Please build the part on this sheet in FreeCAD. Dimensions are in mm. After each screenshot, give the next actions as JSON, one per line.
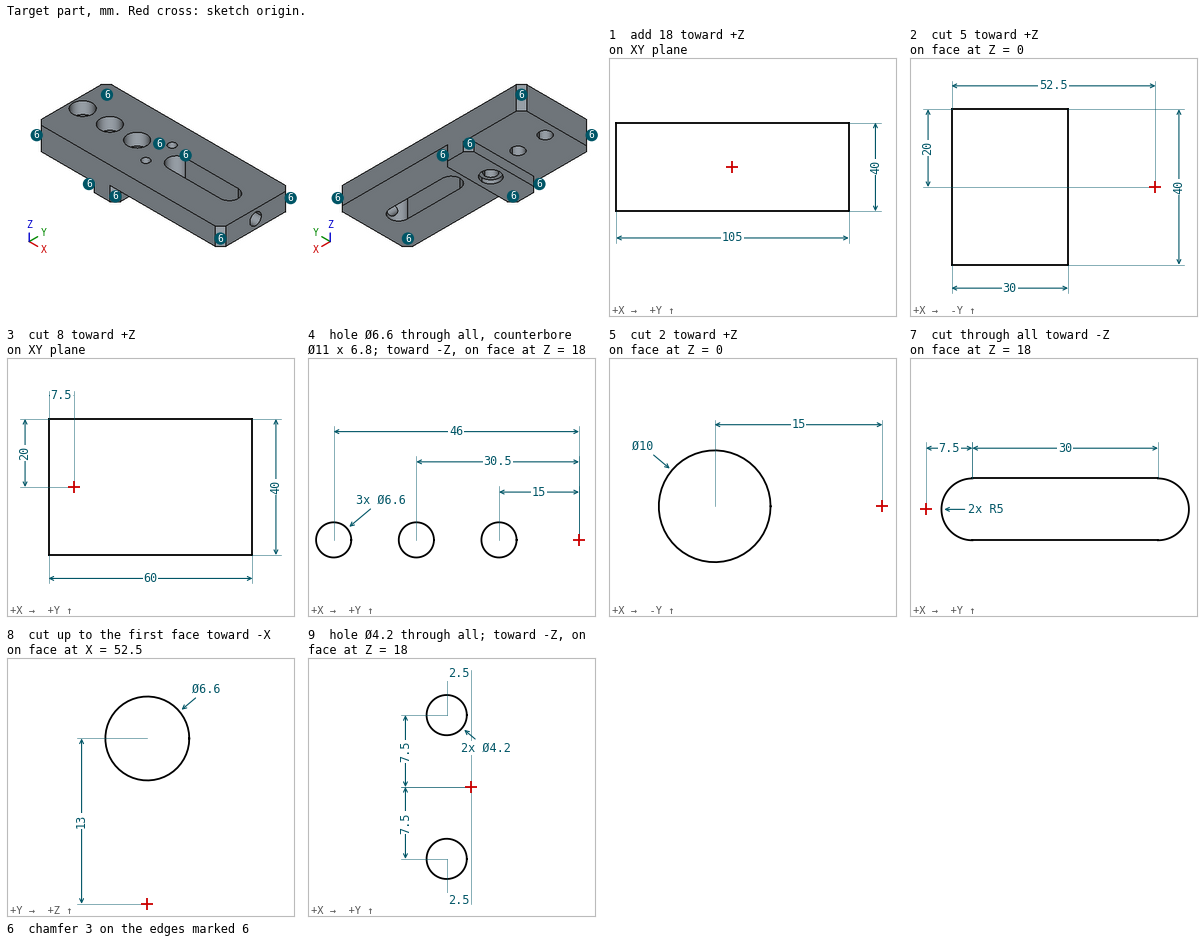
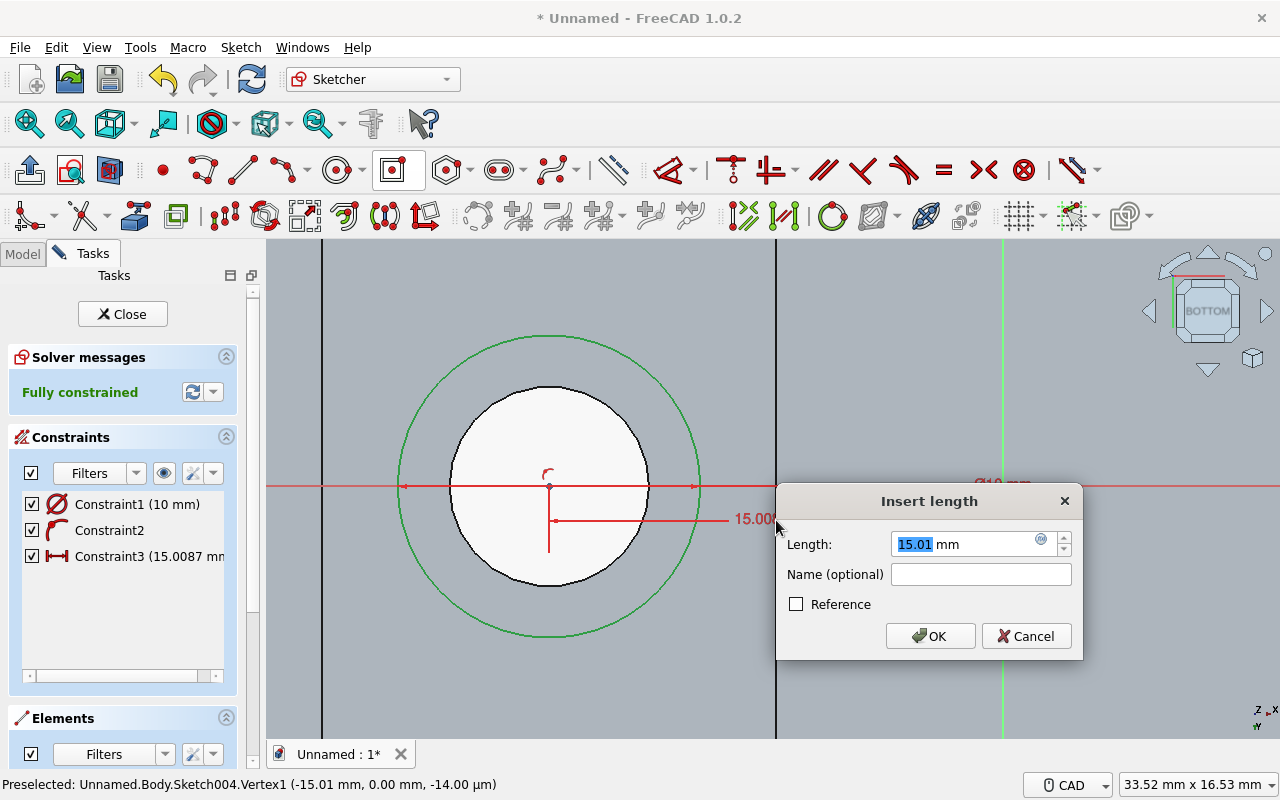
{"action": "type", "text": "15"}
{"action": "key", "text": "Return"}
{"action": "key", "text": "Escape"}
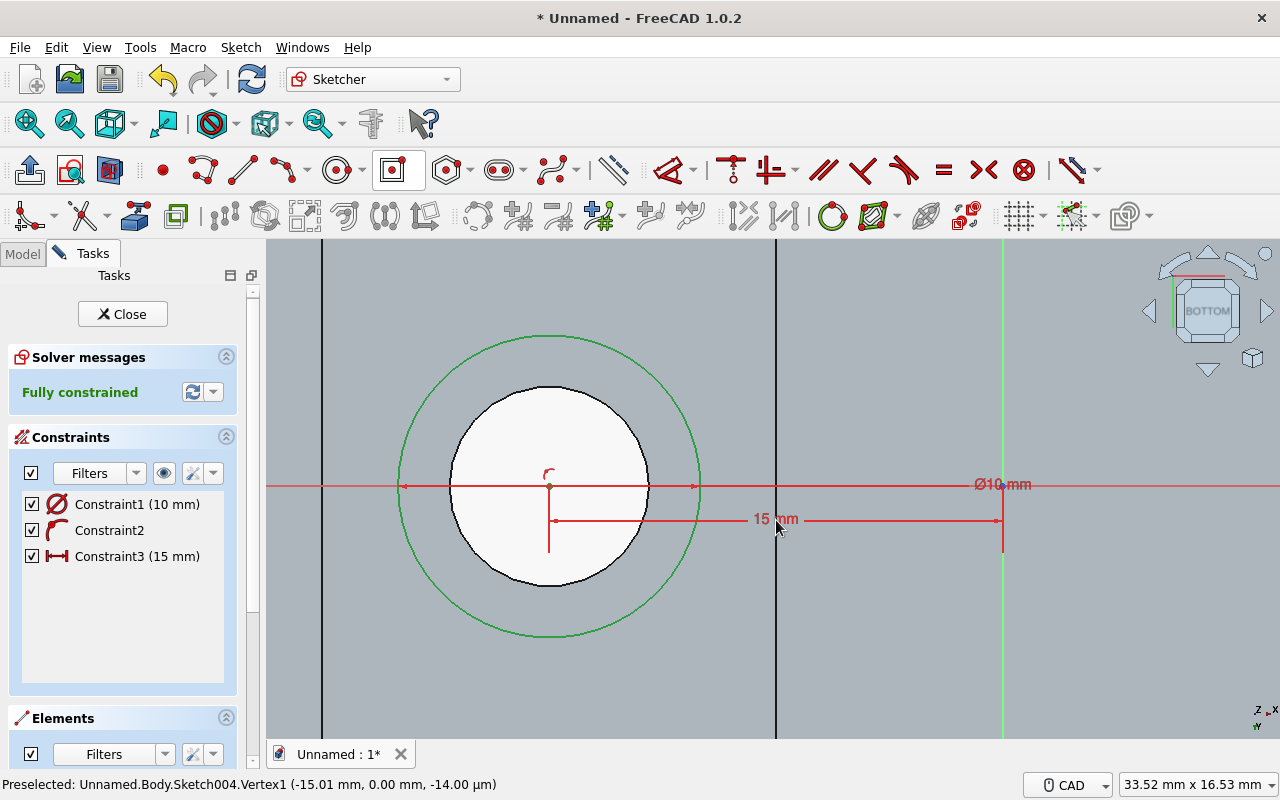
{"action": "left_click", "coordinate": [123, 314]}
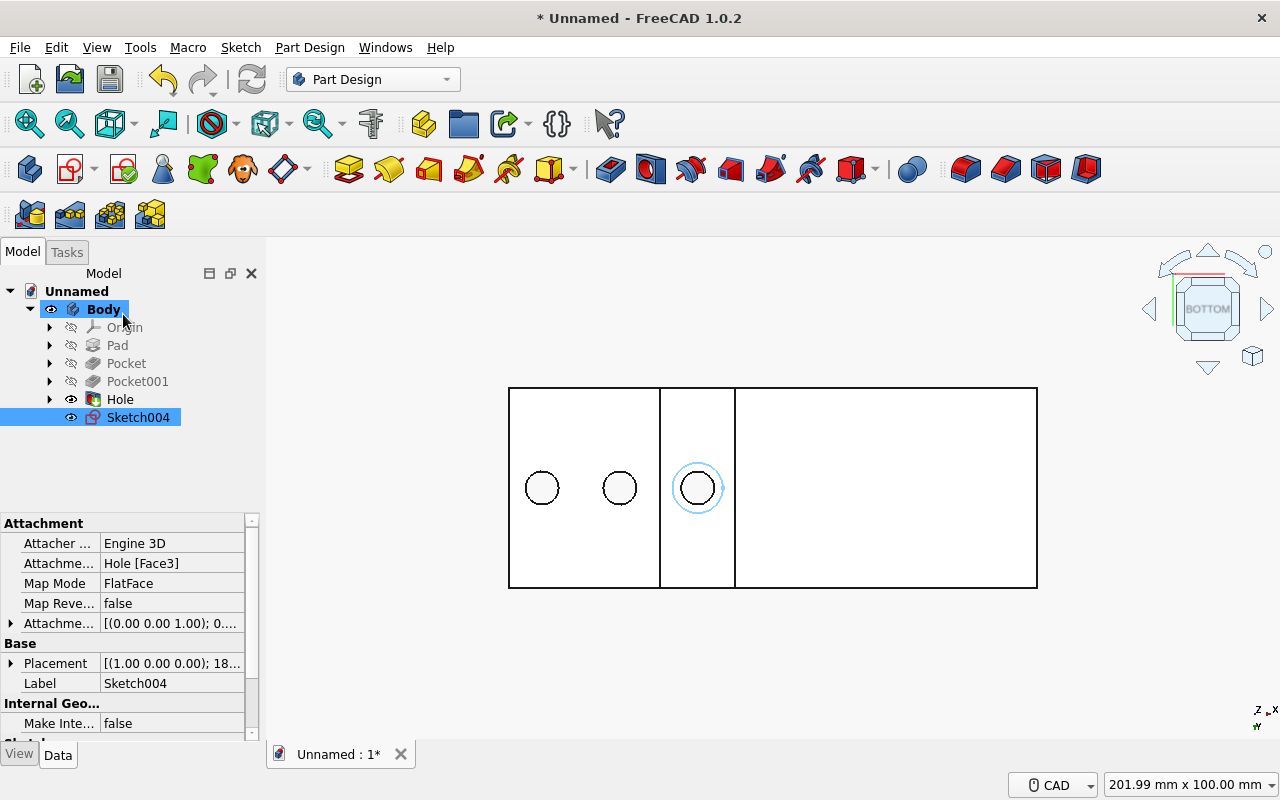
{"action": "left_click", "coordinate": [612, 170]}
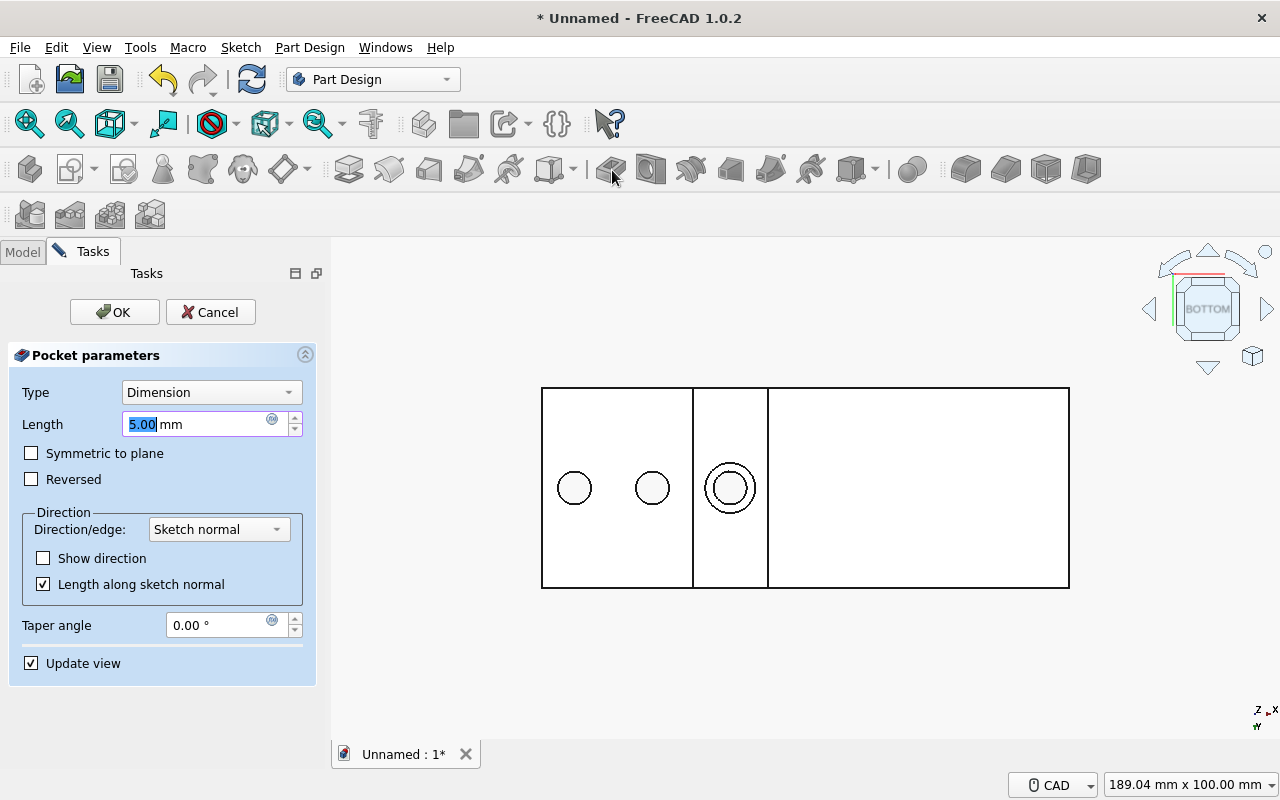
{"action": "type", "text": "2"}
{"action": "key", "text": "Tab"}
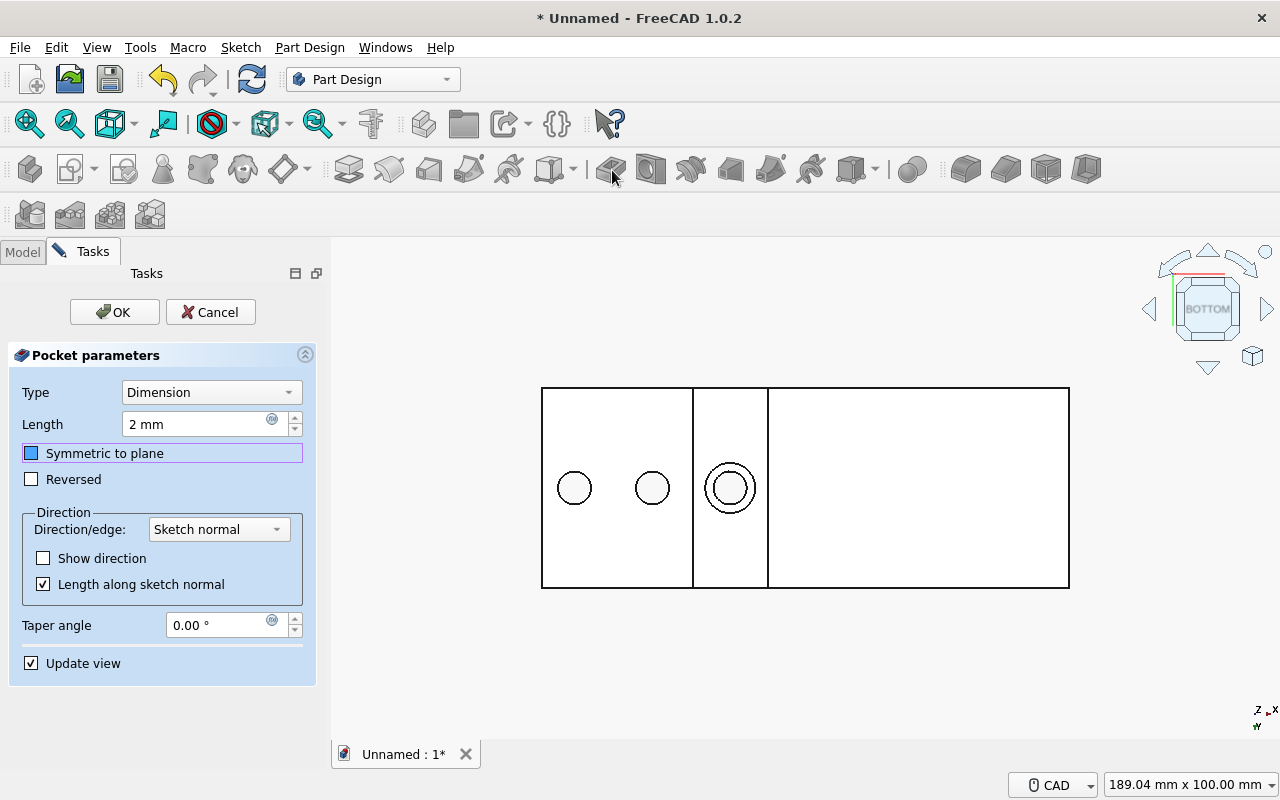
{"action": "left_click", "coordinate": [115, 312]}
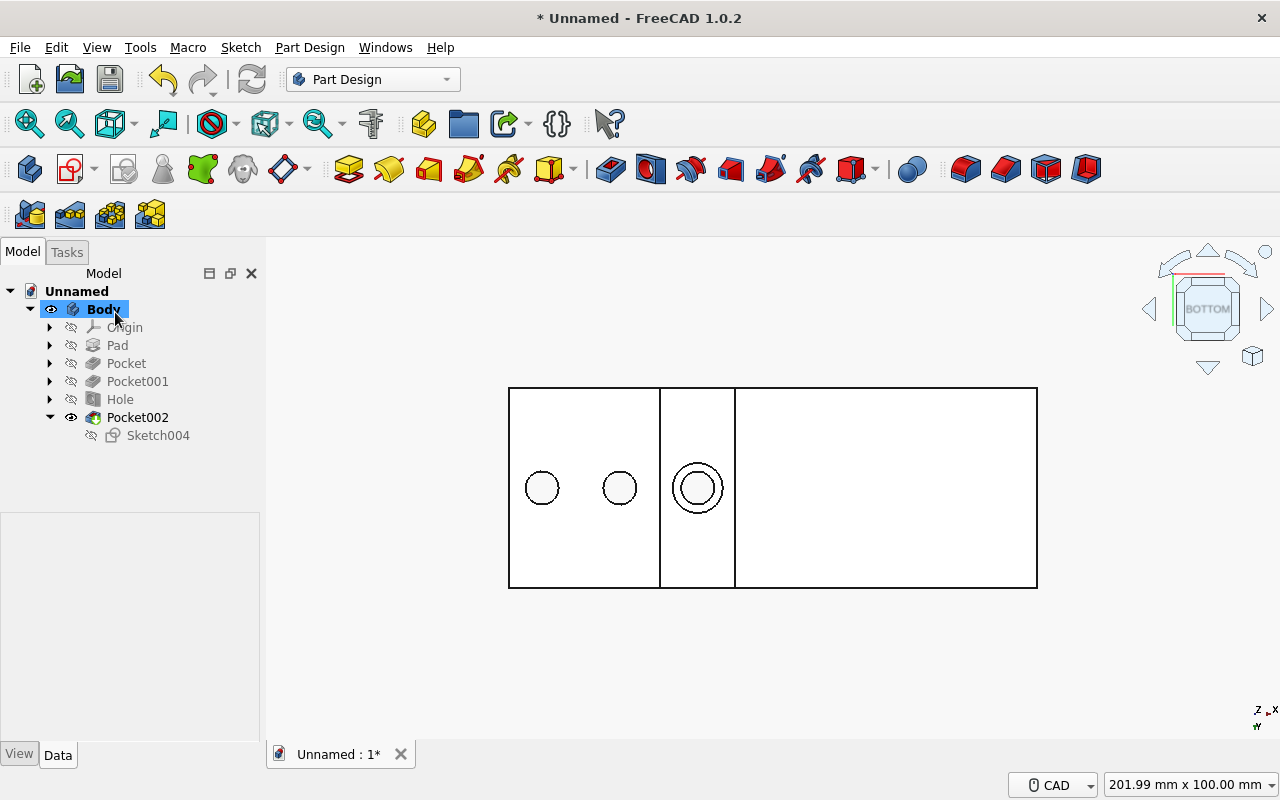
{"action": "key", "text": "0"}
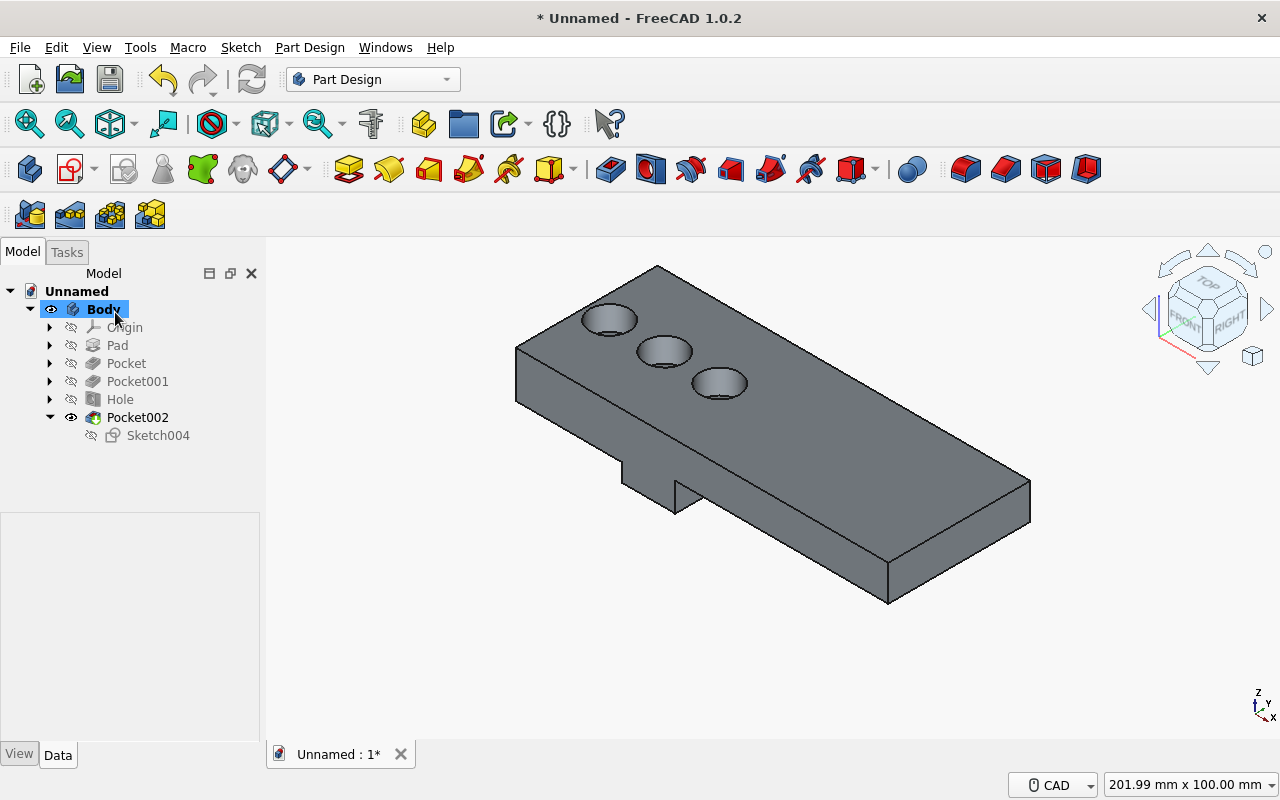
{"action": "left_click", "coordinate": [675, 496]}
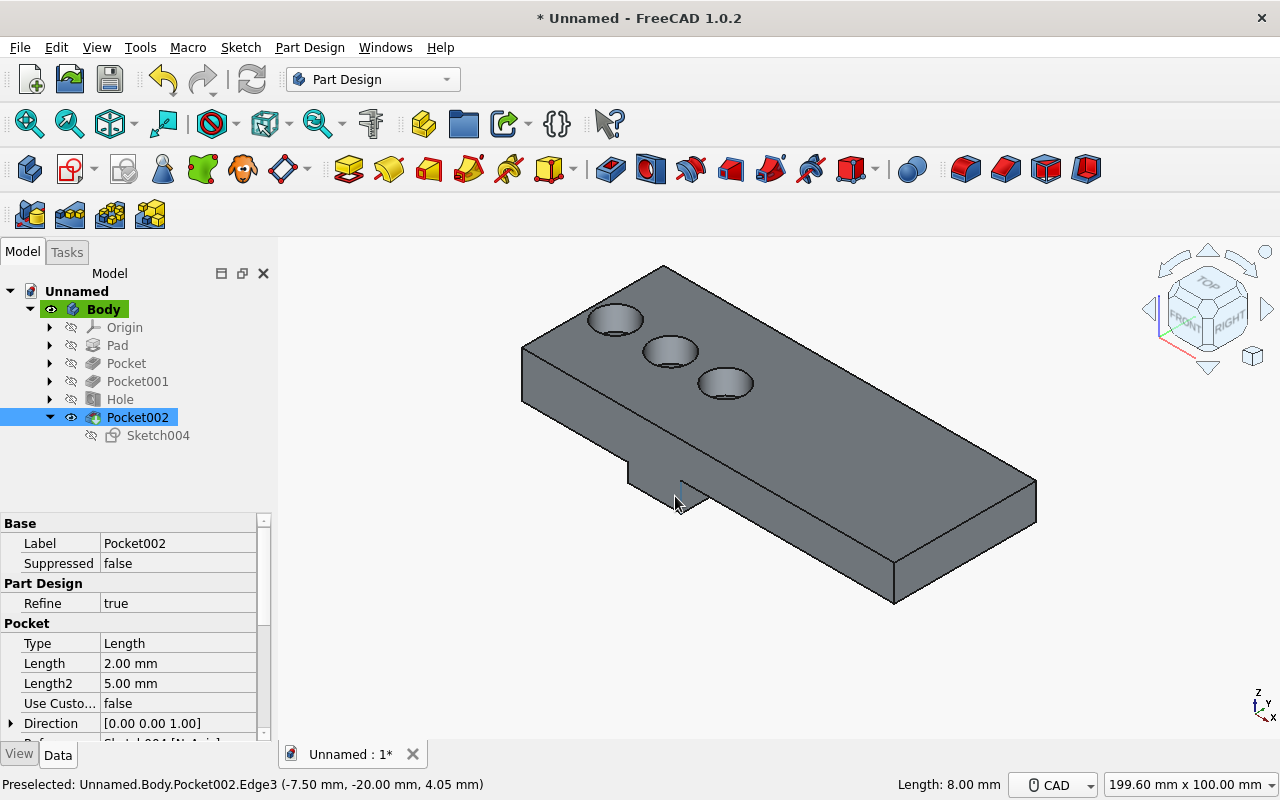
{"action": "left_click", "coordinate": [894, 582], "text": "ctrl"}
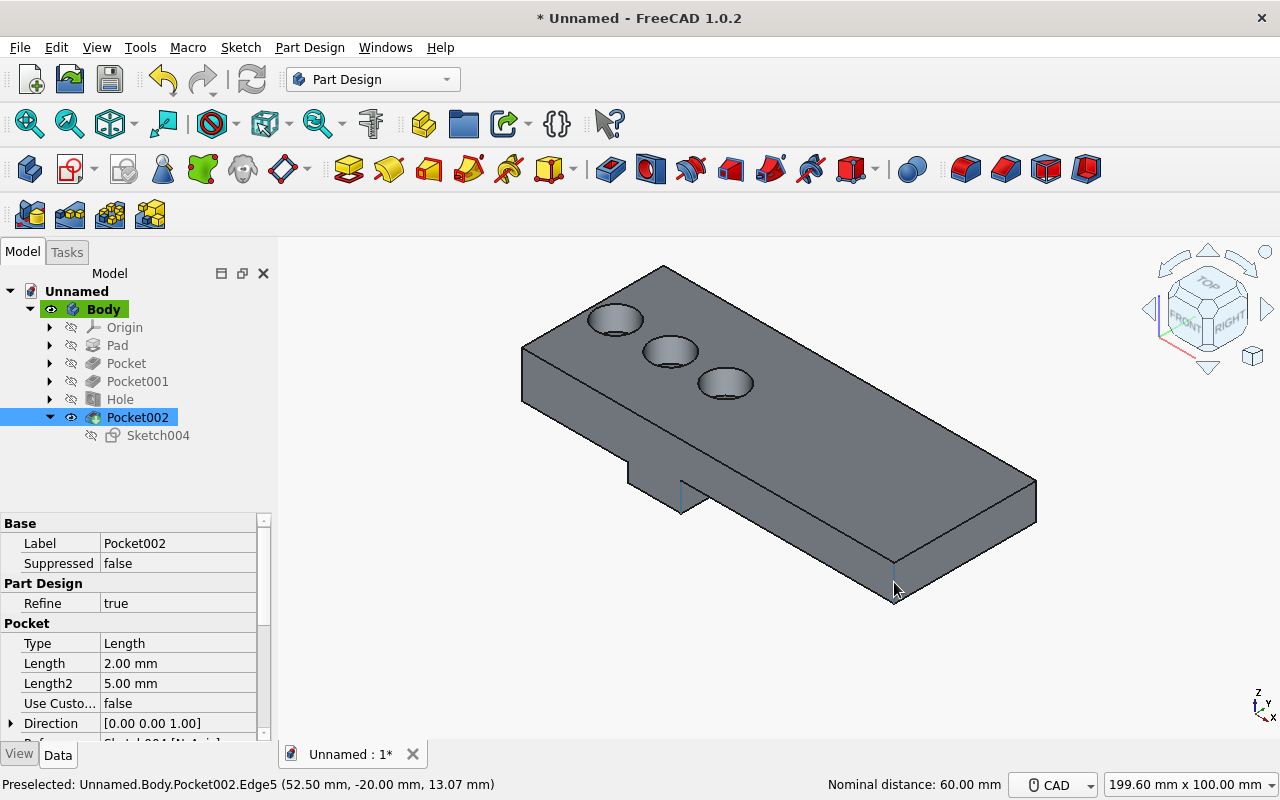
{"action": "key", "text": "2"}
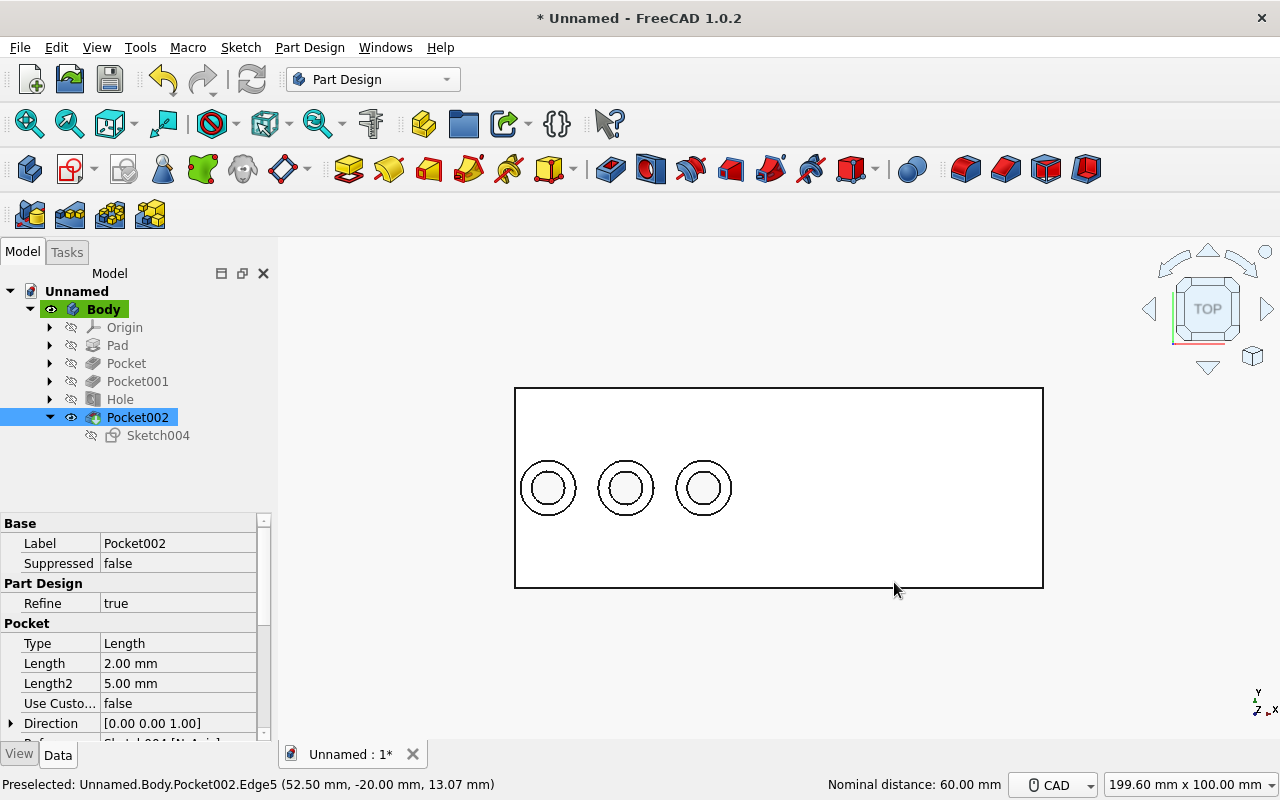
{"action": "key", "text": "1"}